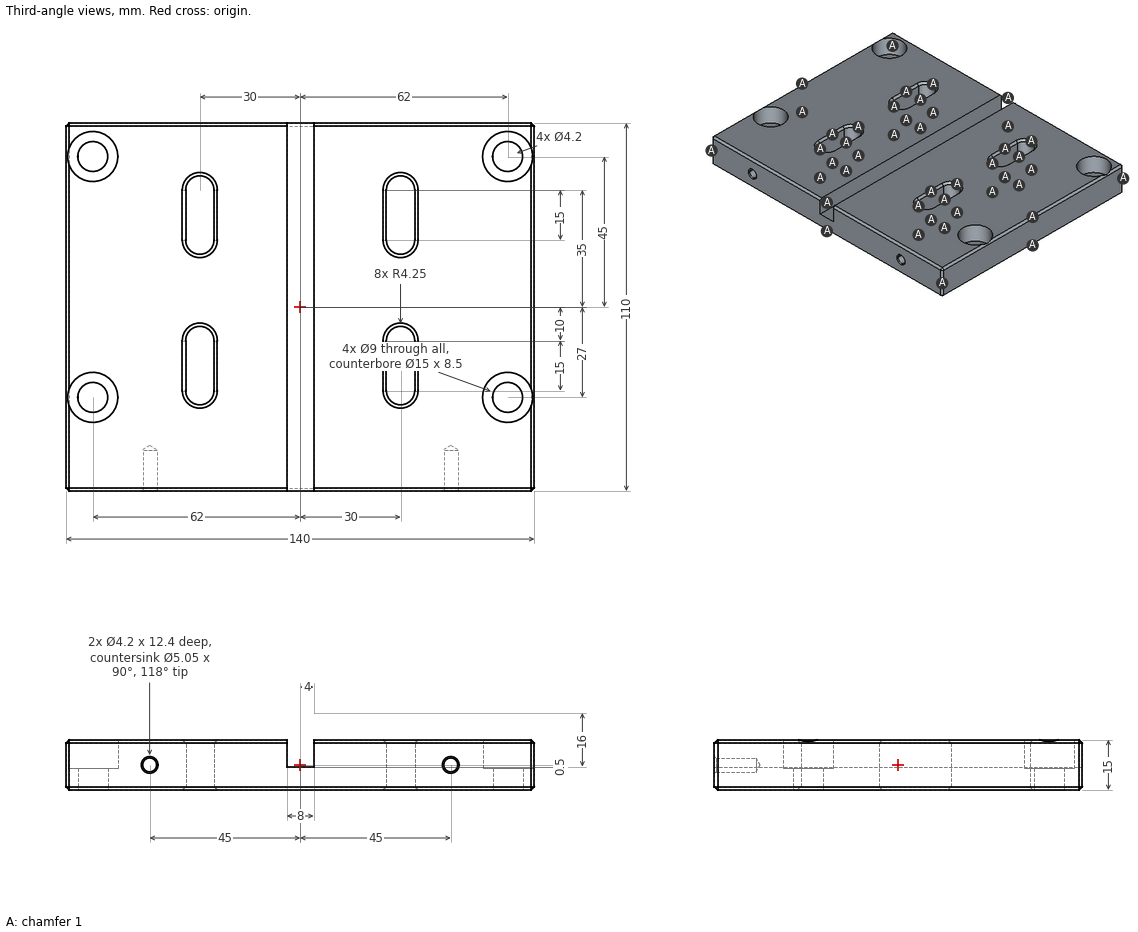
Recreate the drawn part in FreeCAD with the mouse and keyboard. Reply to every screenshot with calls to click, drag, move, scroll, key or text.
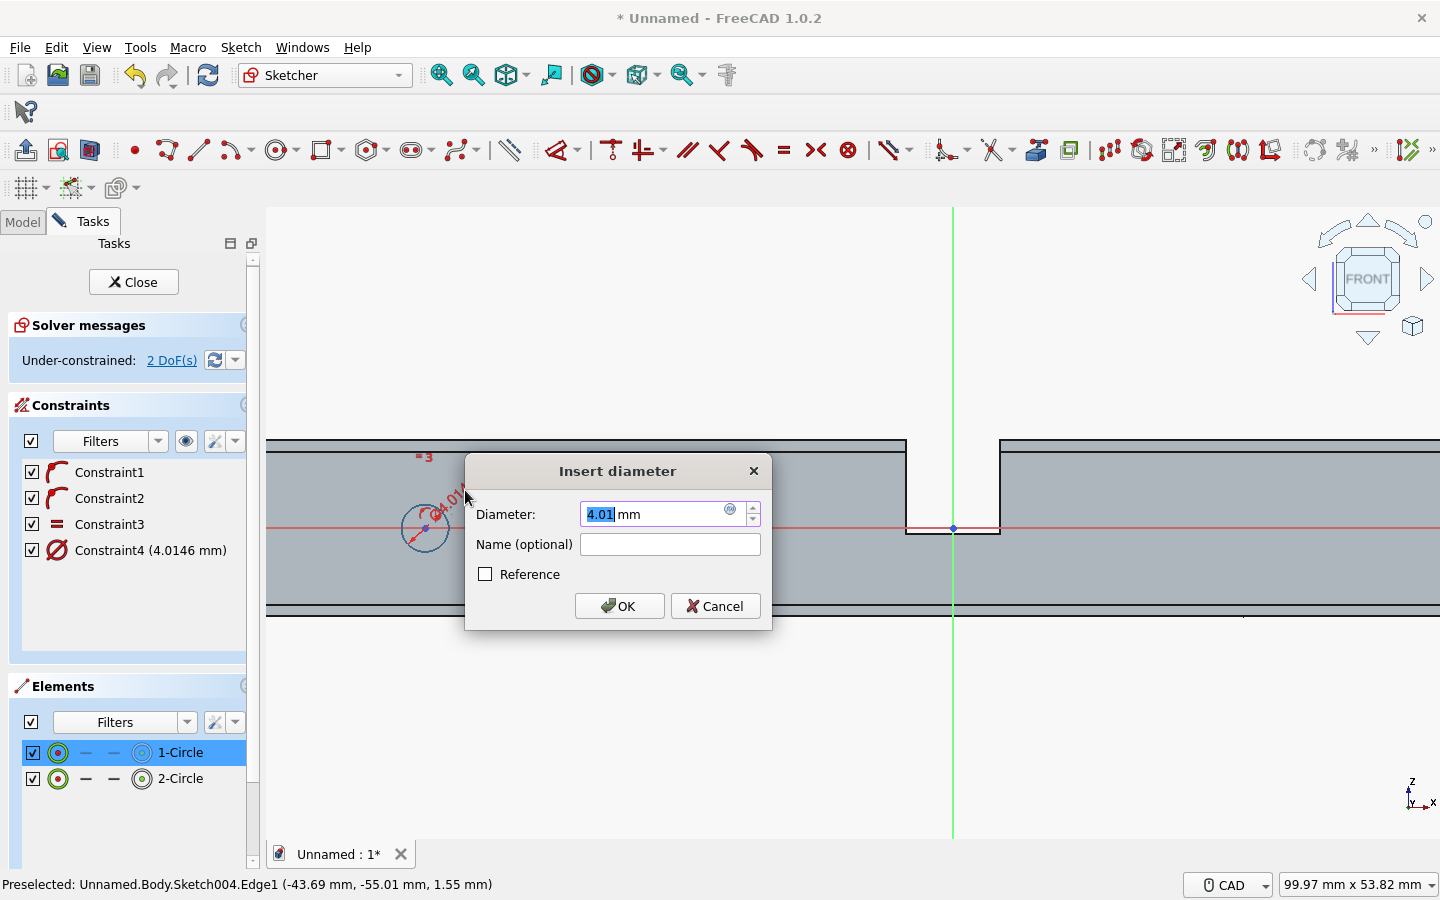
text(4.2)
key(Return)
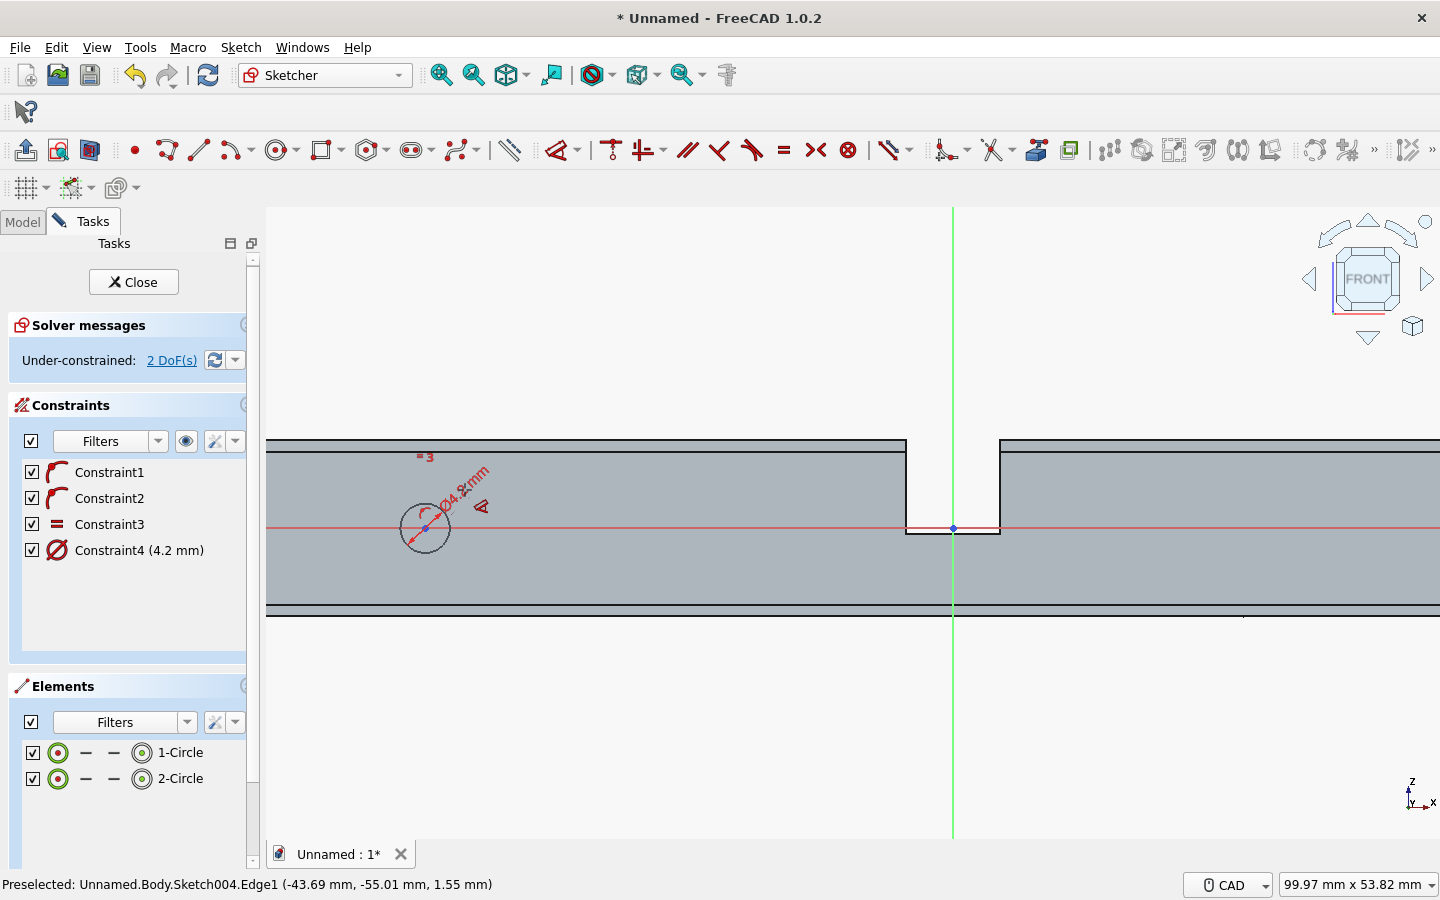
click(425, 528)
click(689, 562)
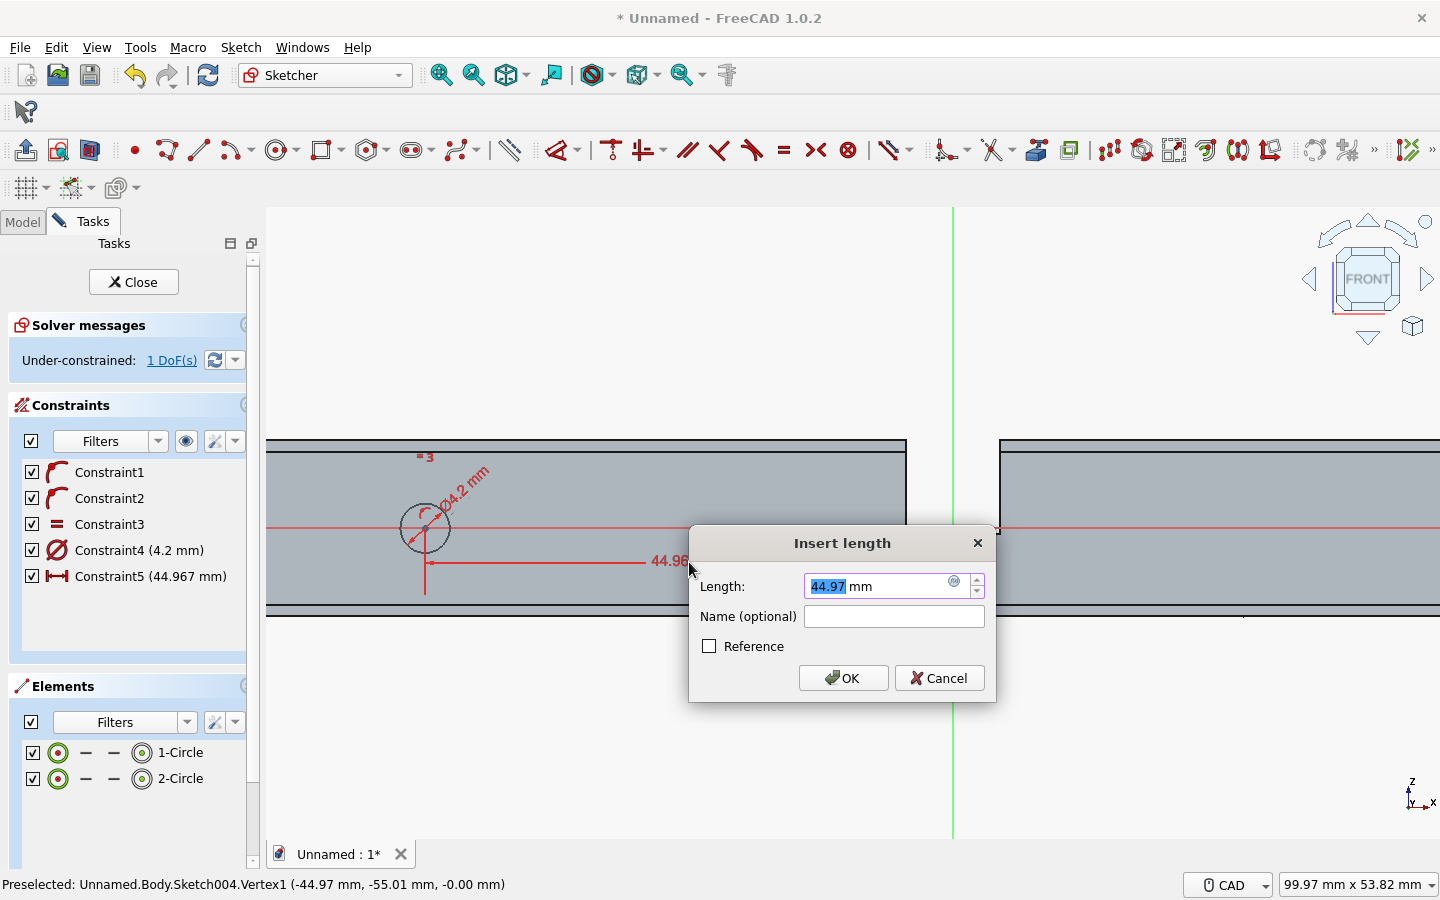
text(45)
key(Return)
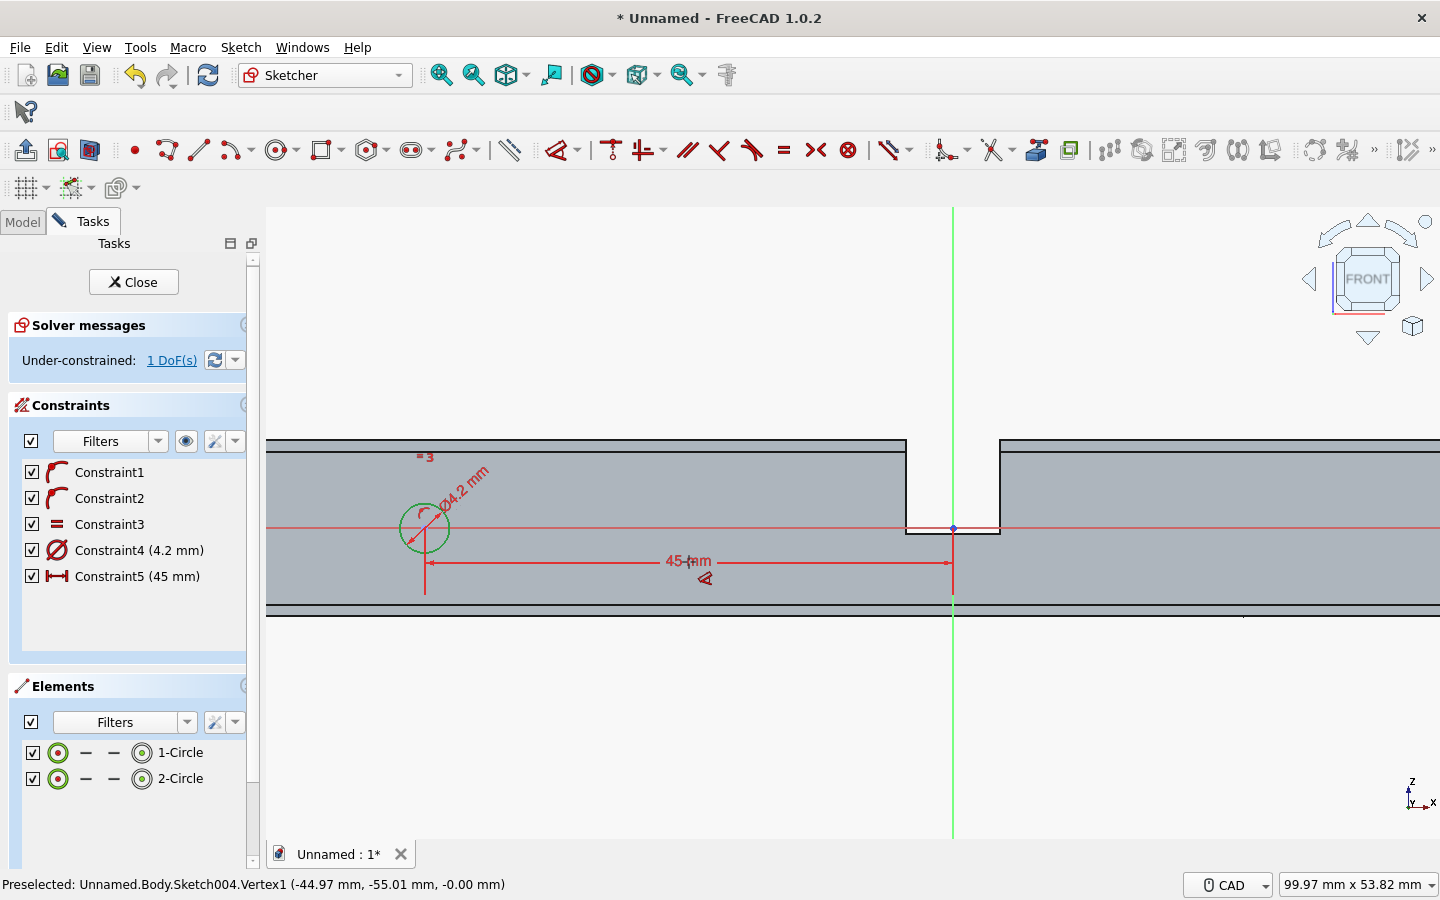
scroll(442, 512, down, 2)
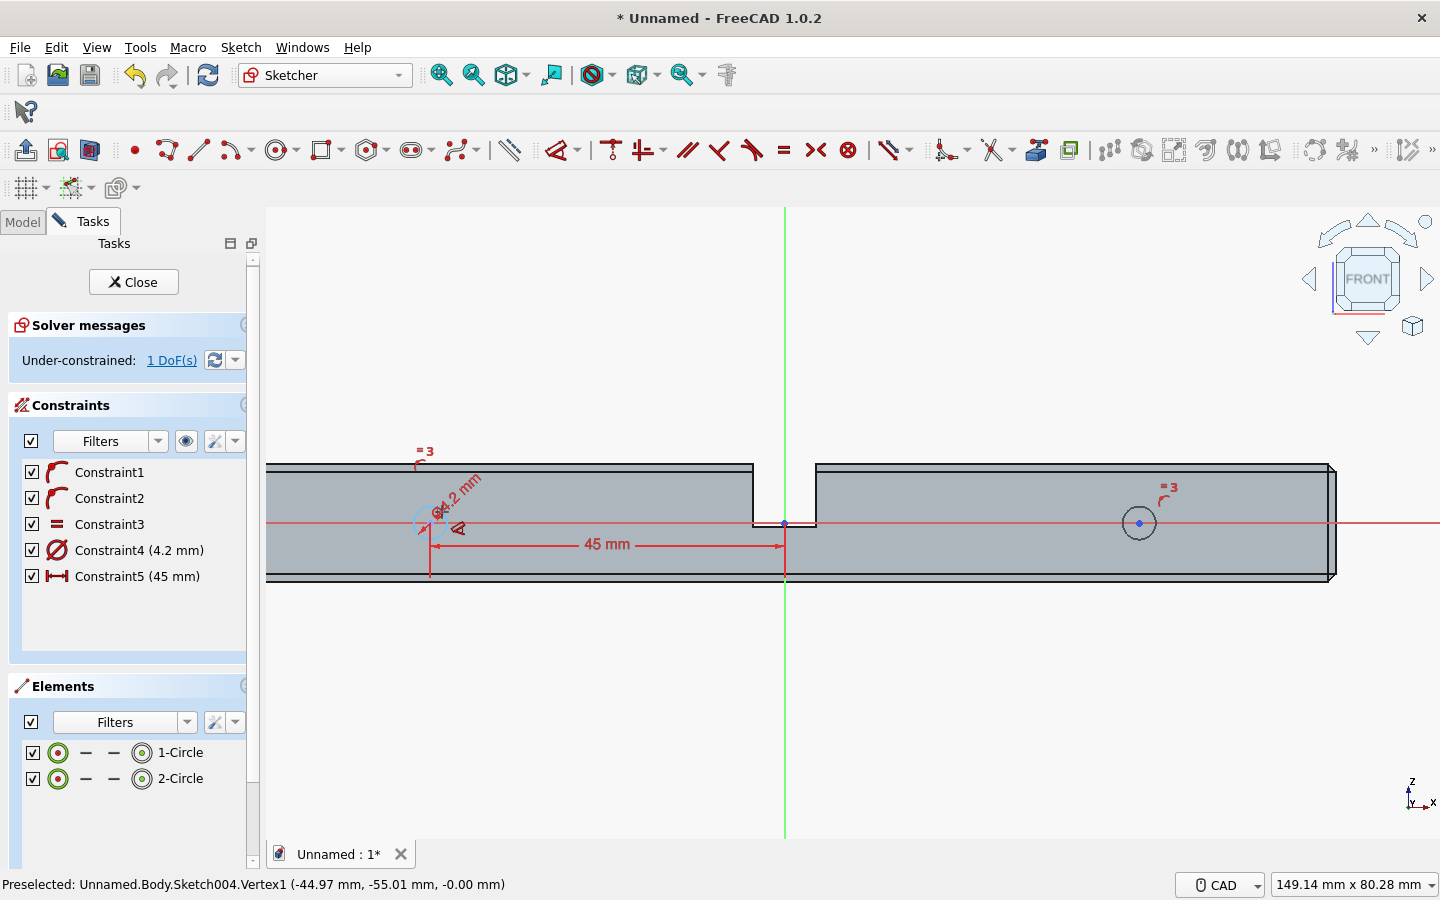
click(1139, 523)
click(962, 557)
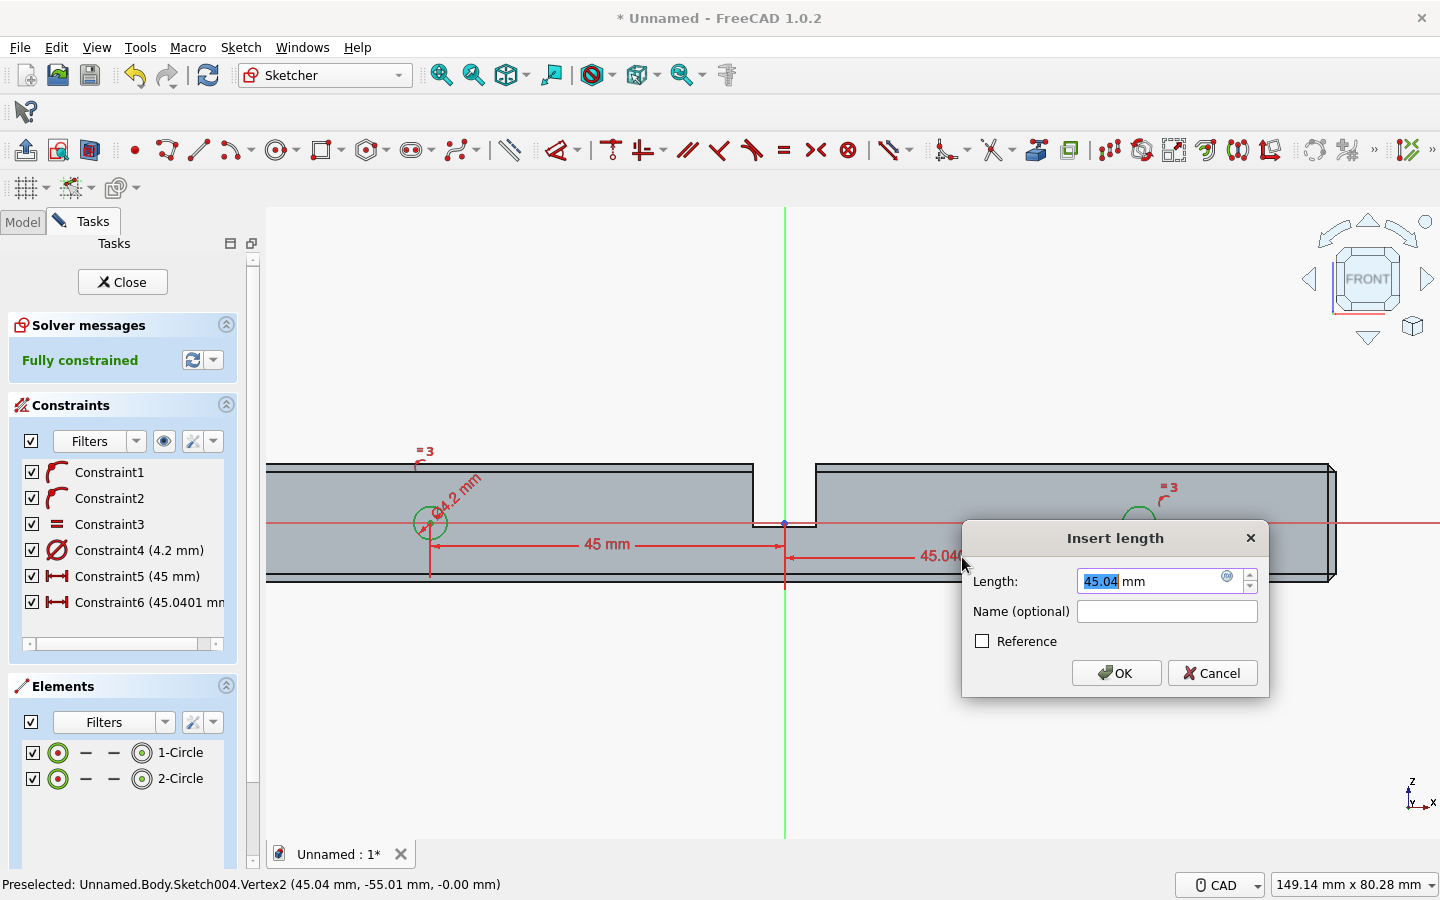
text(45)
key(Return)
key(Escape)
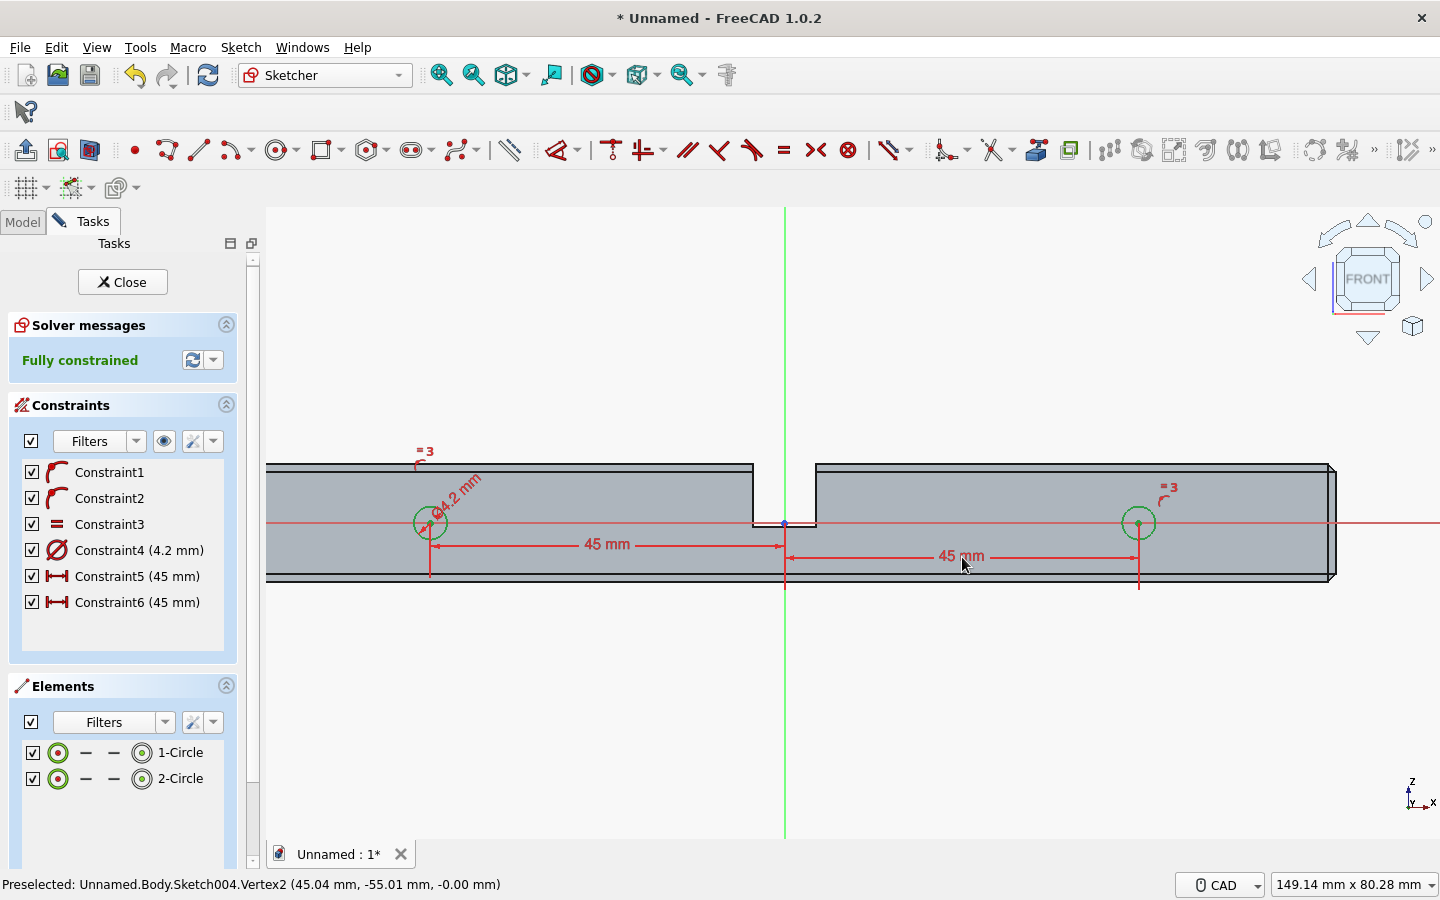
click(123, 282)